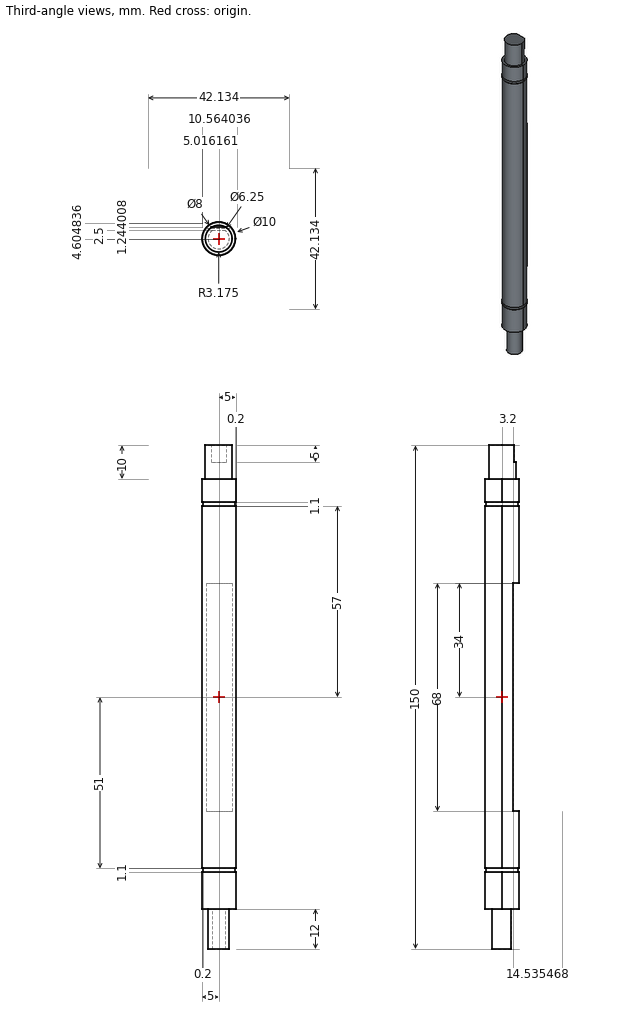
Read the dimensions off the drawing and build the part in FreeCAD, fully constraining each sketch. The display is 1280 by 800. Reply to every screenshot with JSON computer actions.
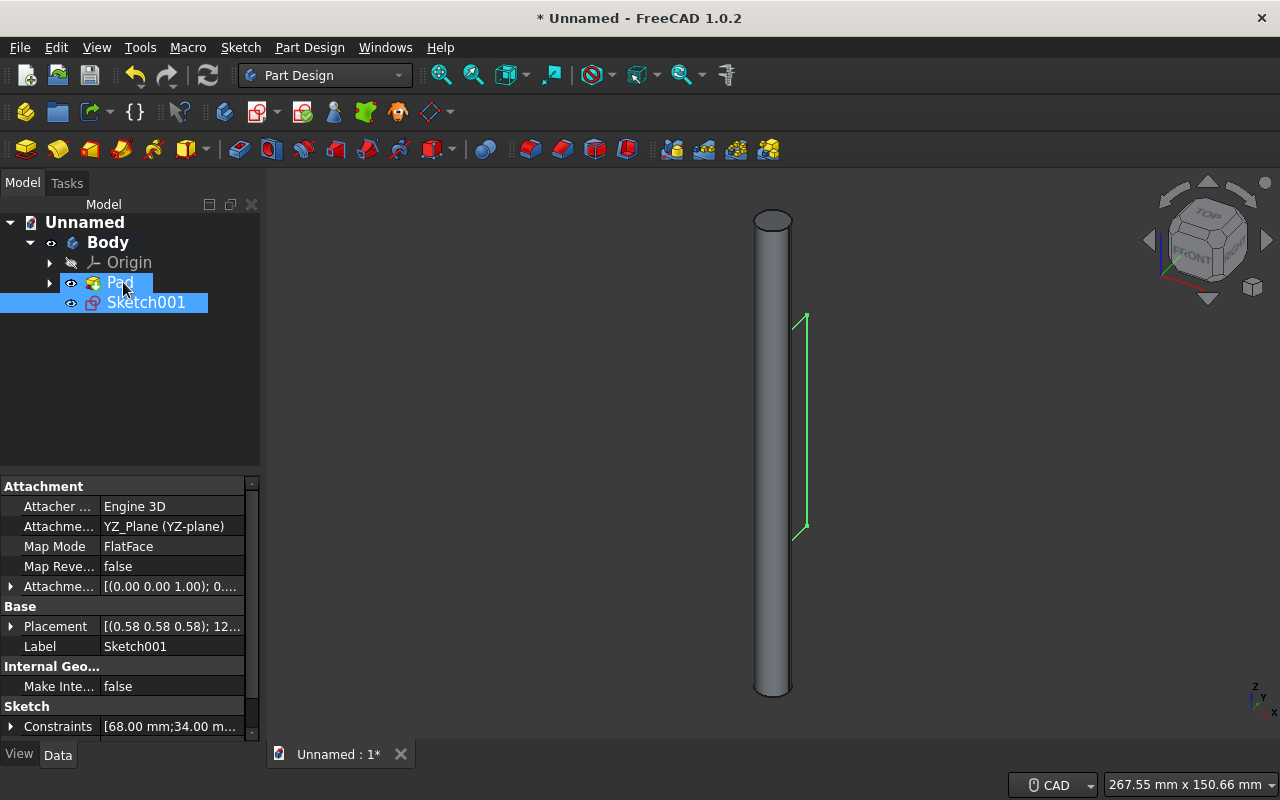
{"action": "left_click", "coordinate": [240, 150]}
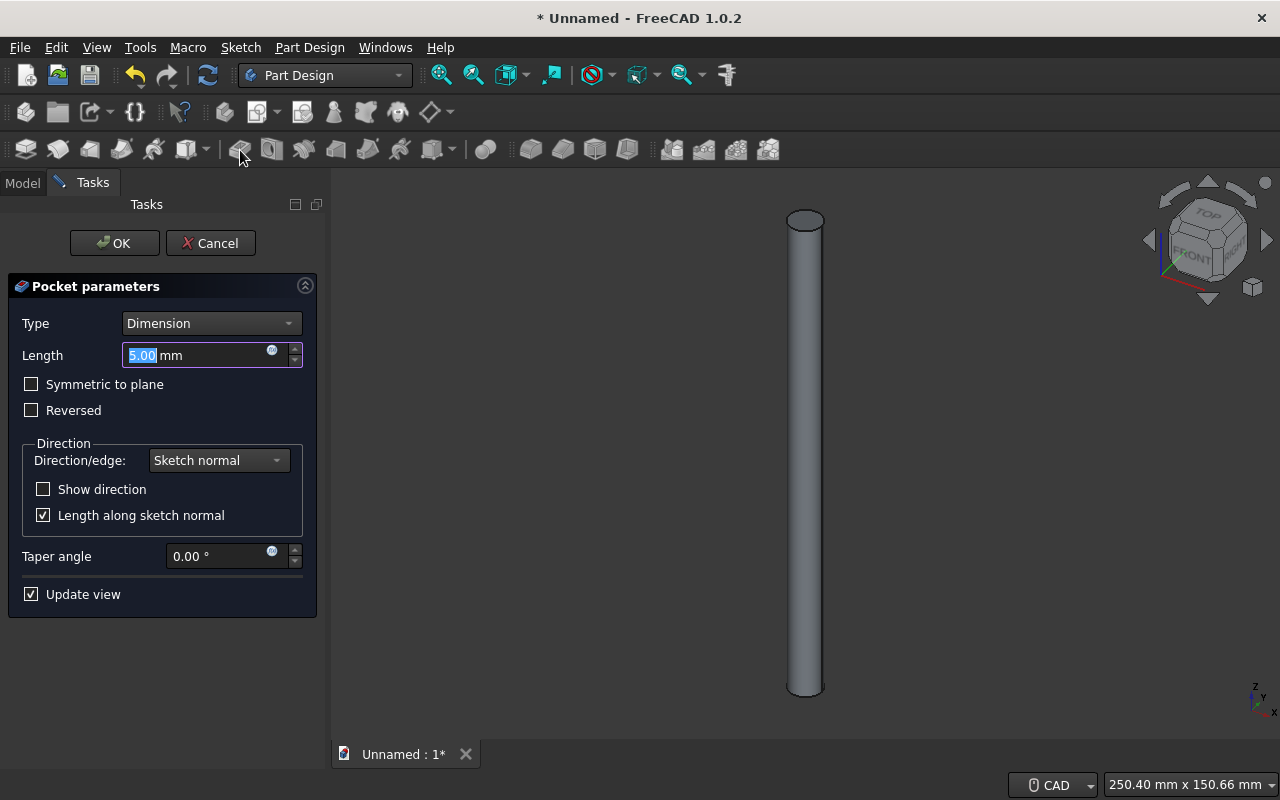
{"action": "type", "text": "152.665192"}
{"action": "key", "text": "Tab"}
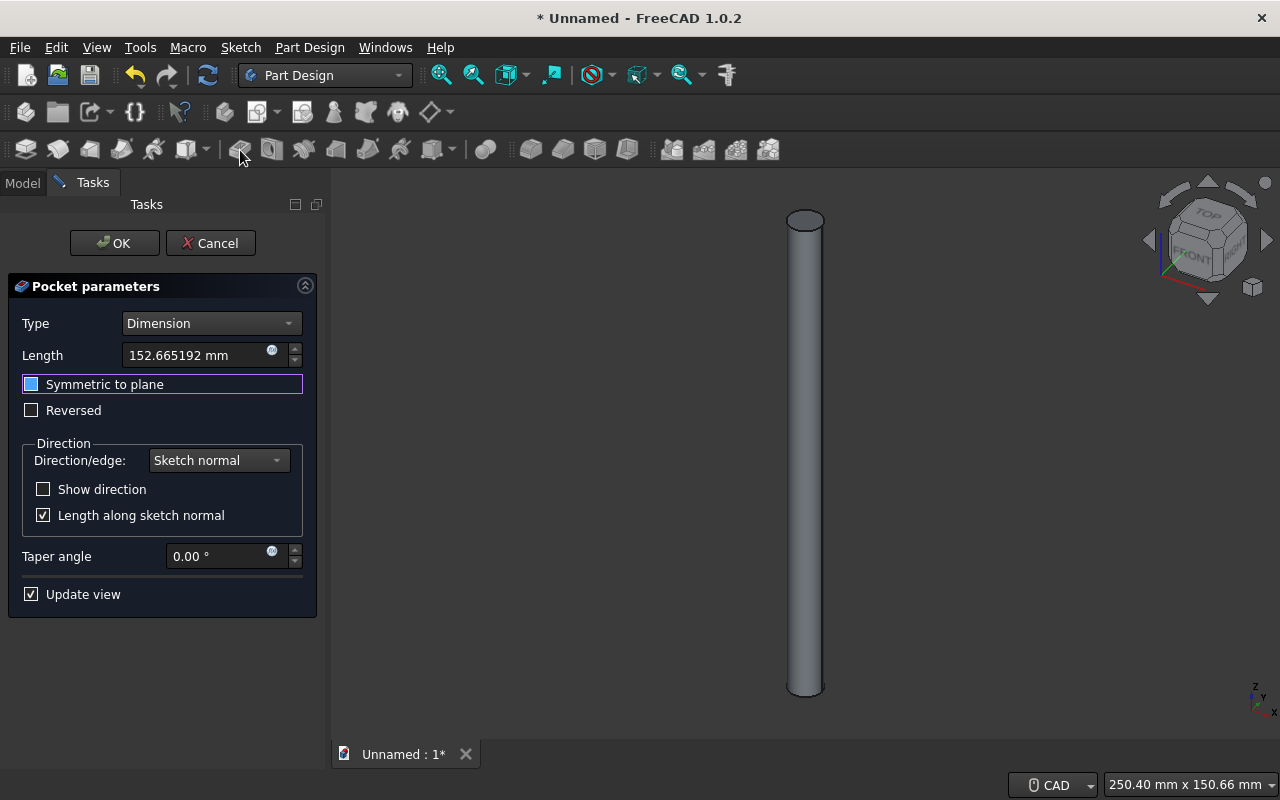
{"action": "left_click", "coordinate": [30, 384]}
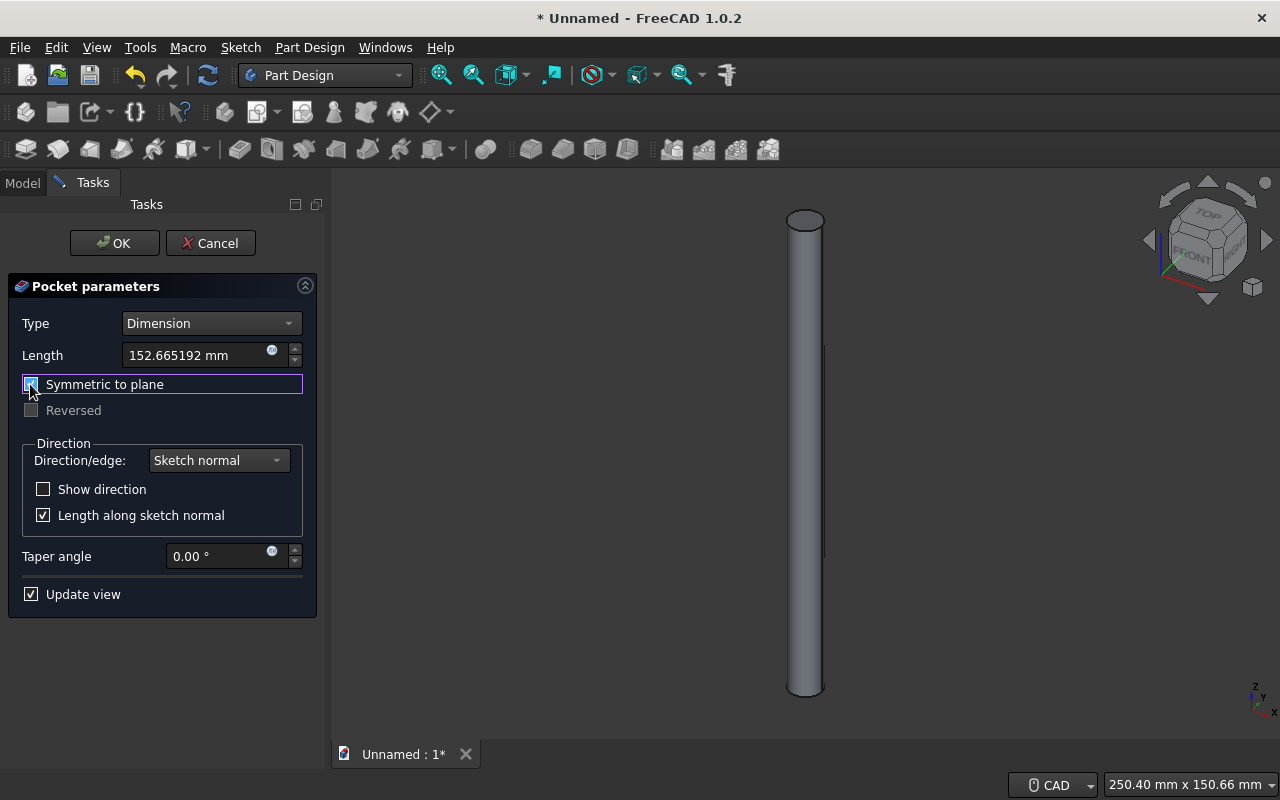
{"action": "left_click", "coordinate": [115, 243]}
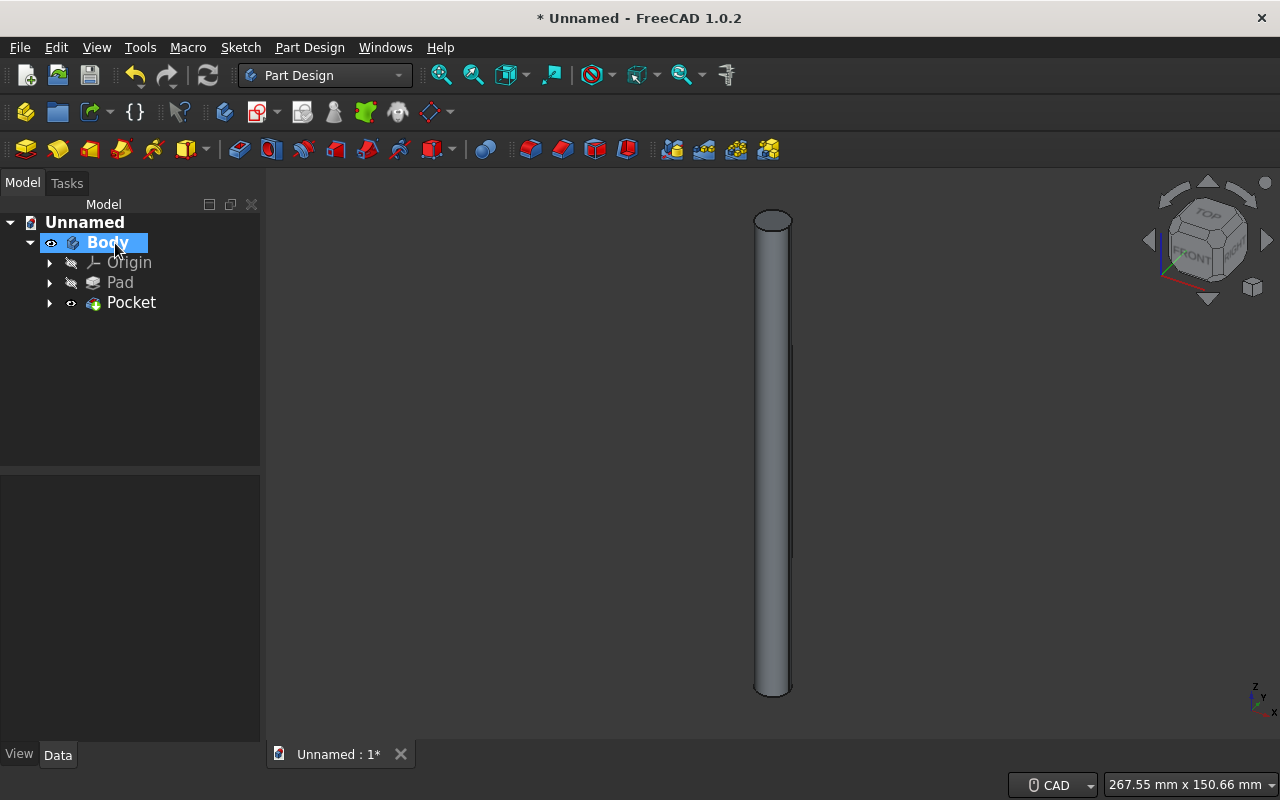
{"action": "left_click", "coordinate": [50, 263]}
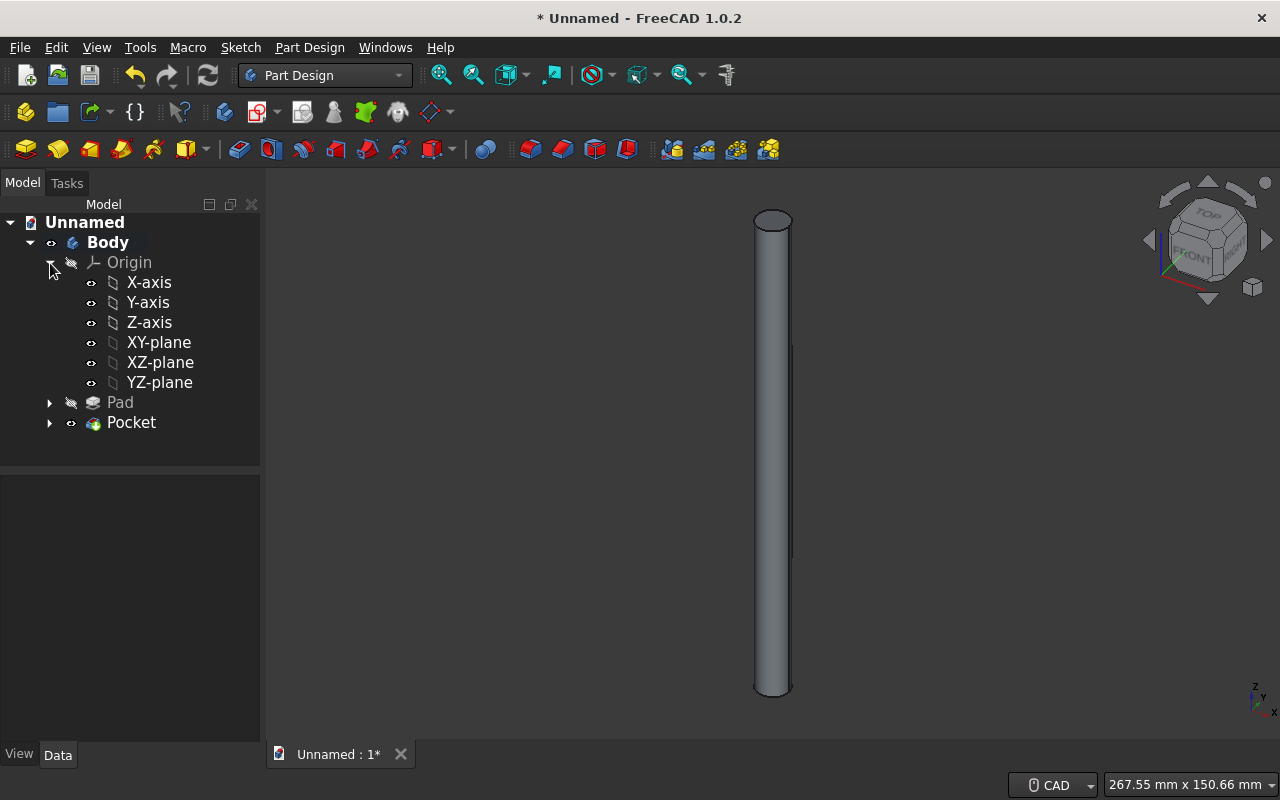
{"action": "left_click", "coordinate": [136, 343]}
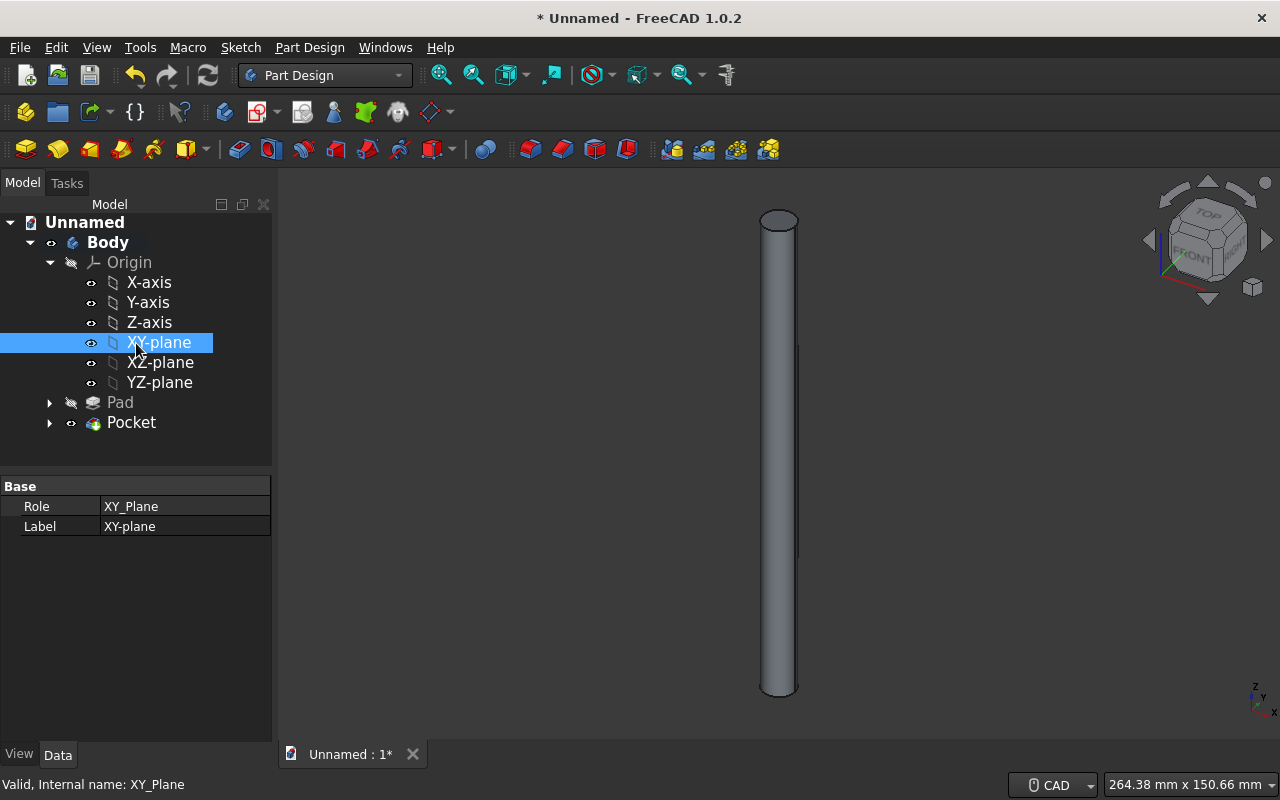
{"action": "left_click", "coordinate": [430, 112]}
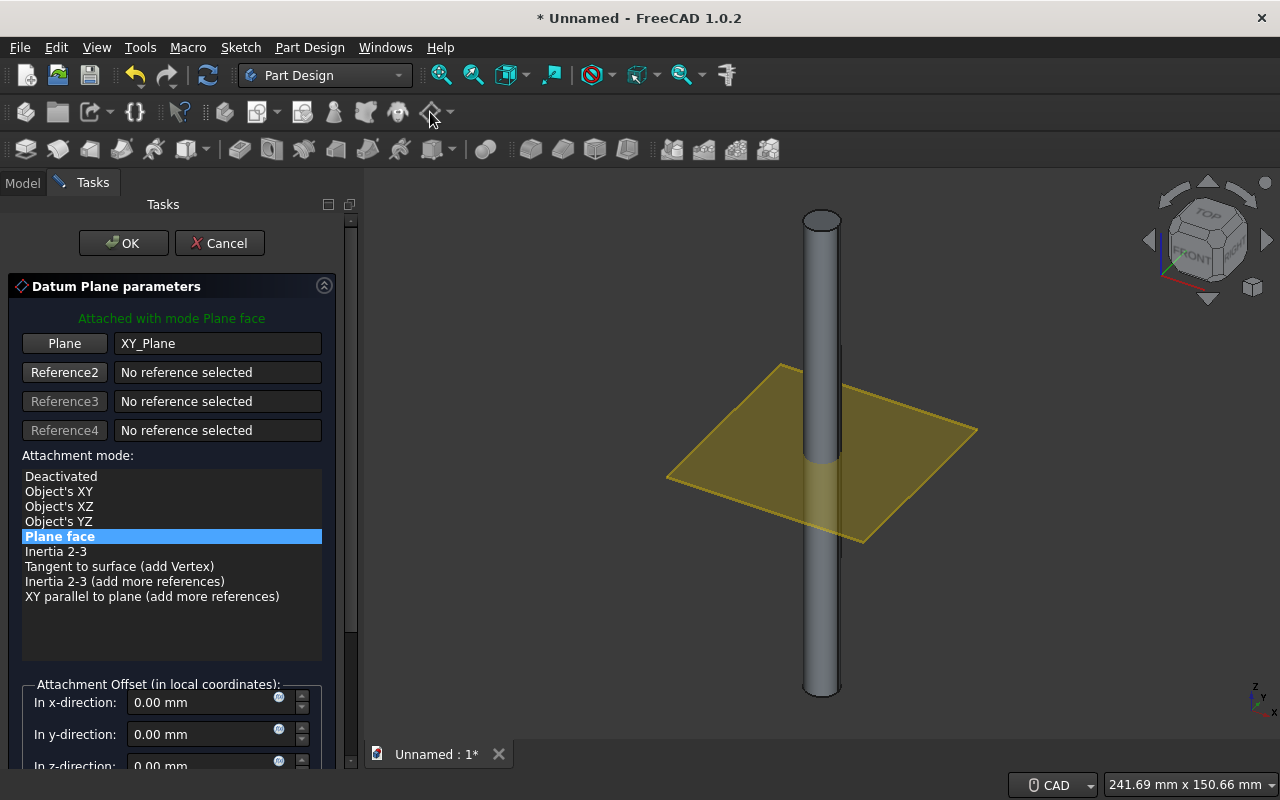
{"action": "scroll", "coordinate": [351, 491], "scroll_direction": "down", "scroll_amount": 2}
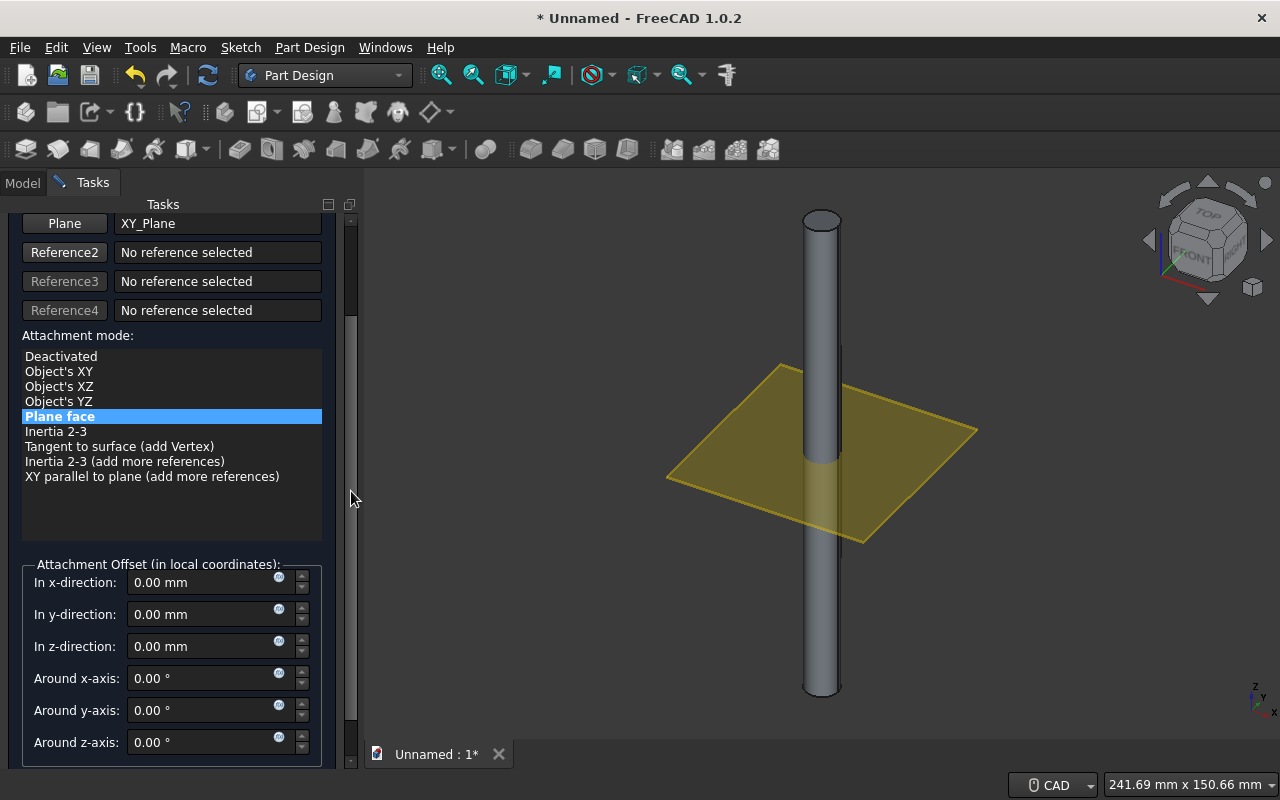
{"action": "triple_click", "coordinate": [210, 646]}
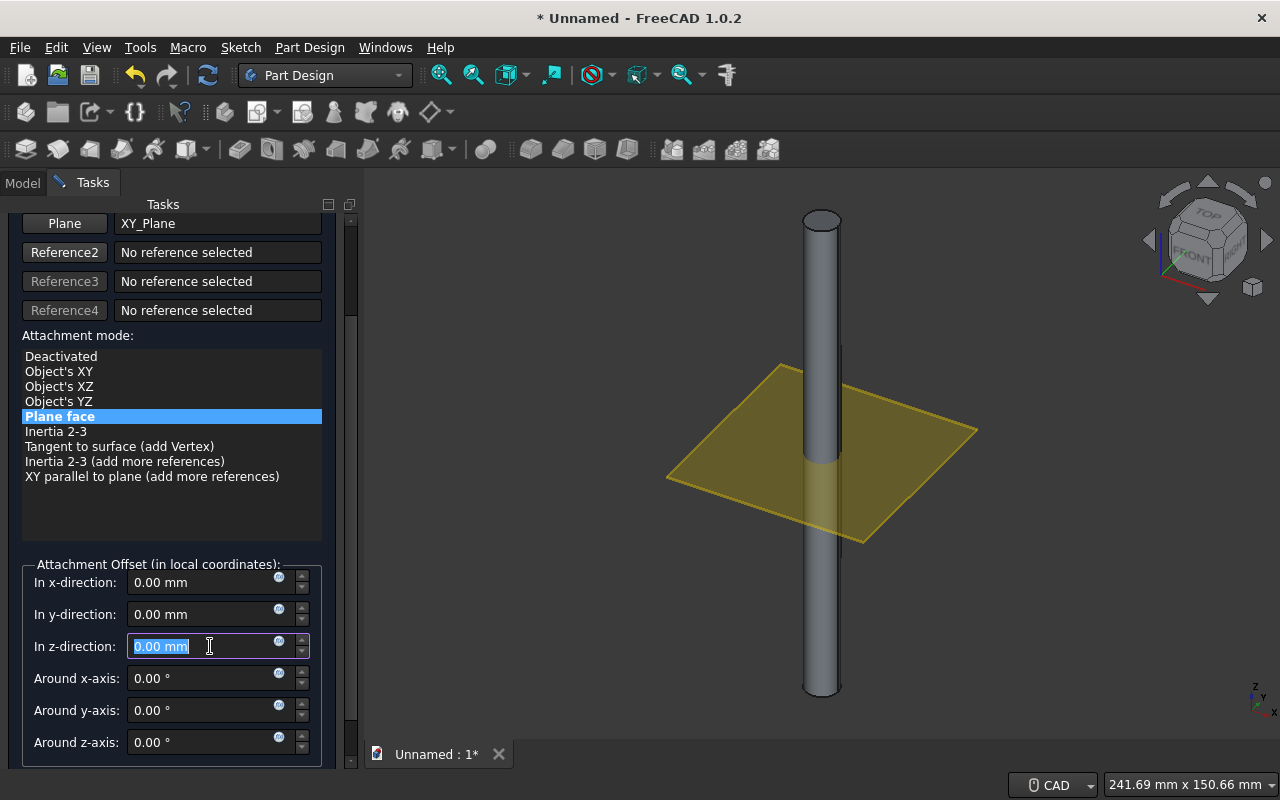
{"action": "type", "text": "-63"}
{"action": "key", "text": "Tab"}